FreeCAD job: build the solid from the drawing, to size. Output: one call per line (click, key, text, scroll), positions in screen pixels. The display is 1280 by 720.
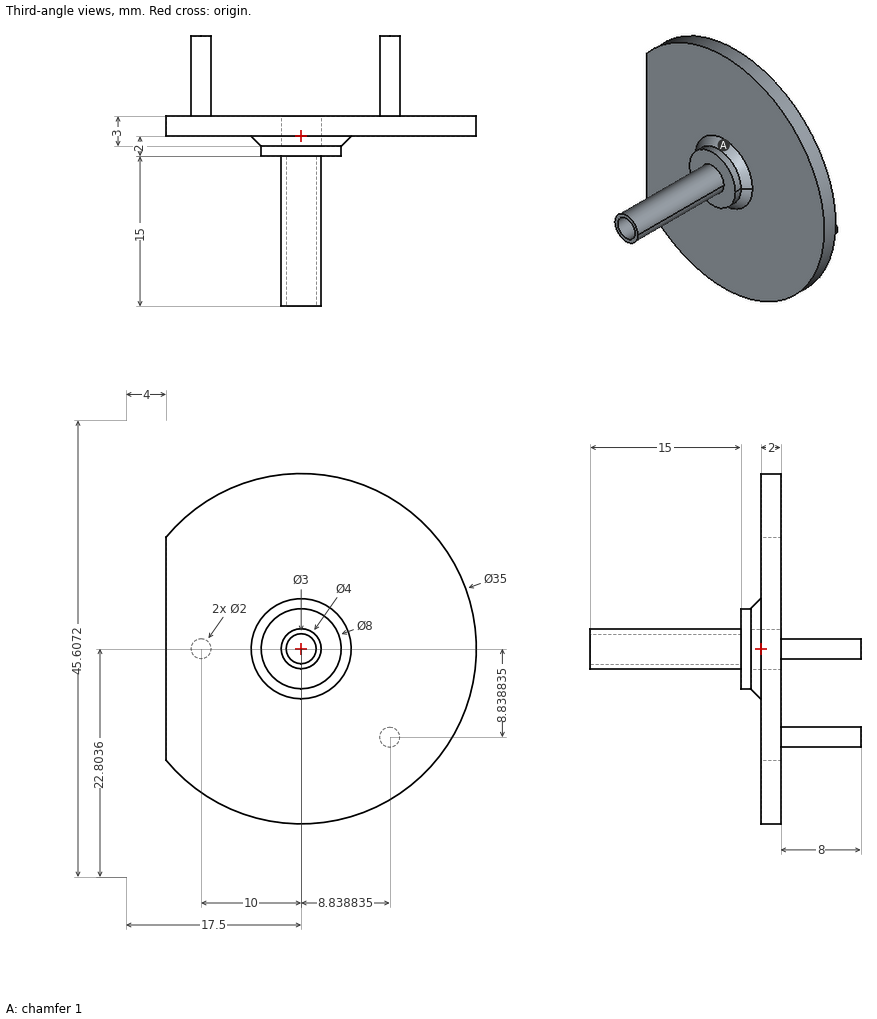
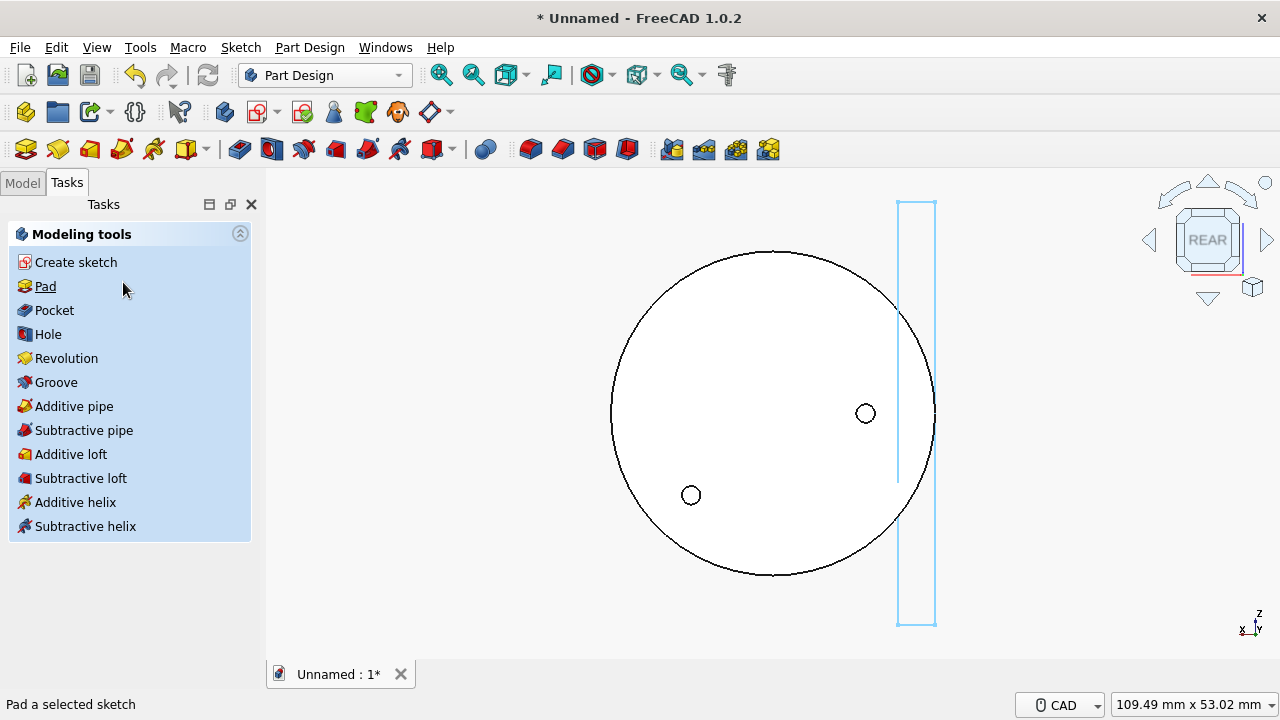
click(240, 150)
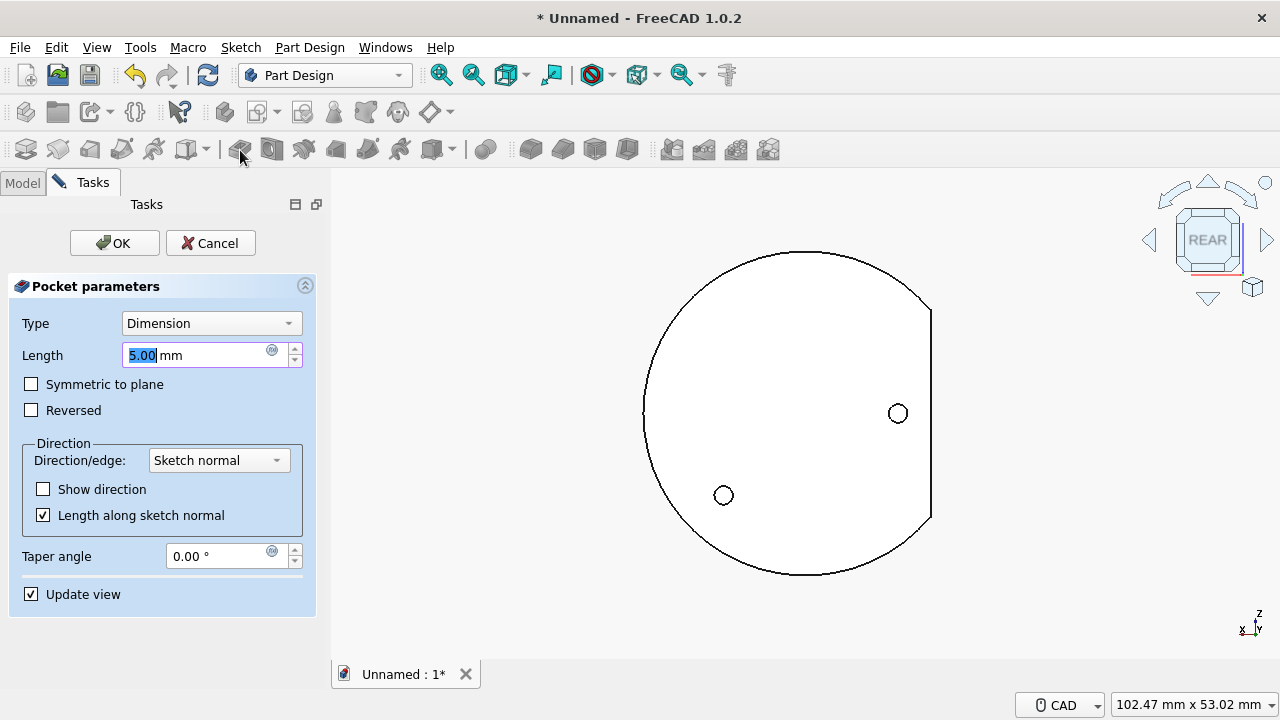
click(212, 324)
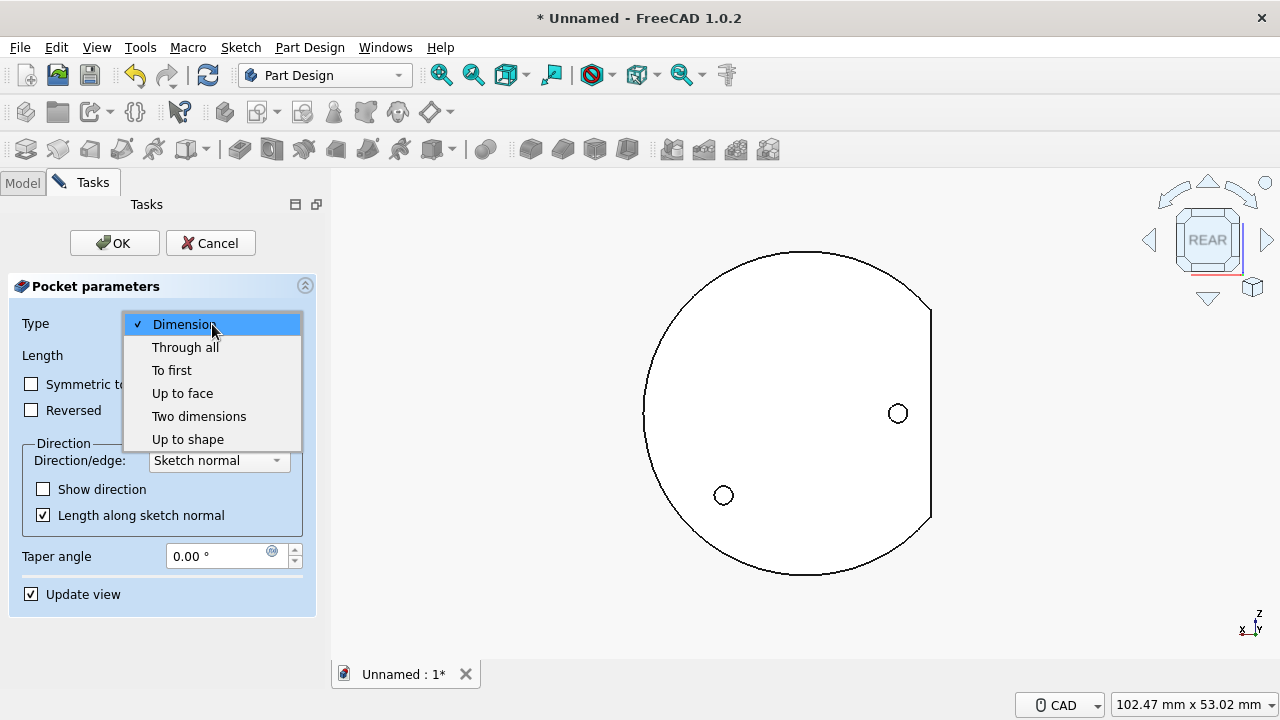
click(212, 348)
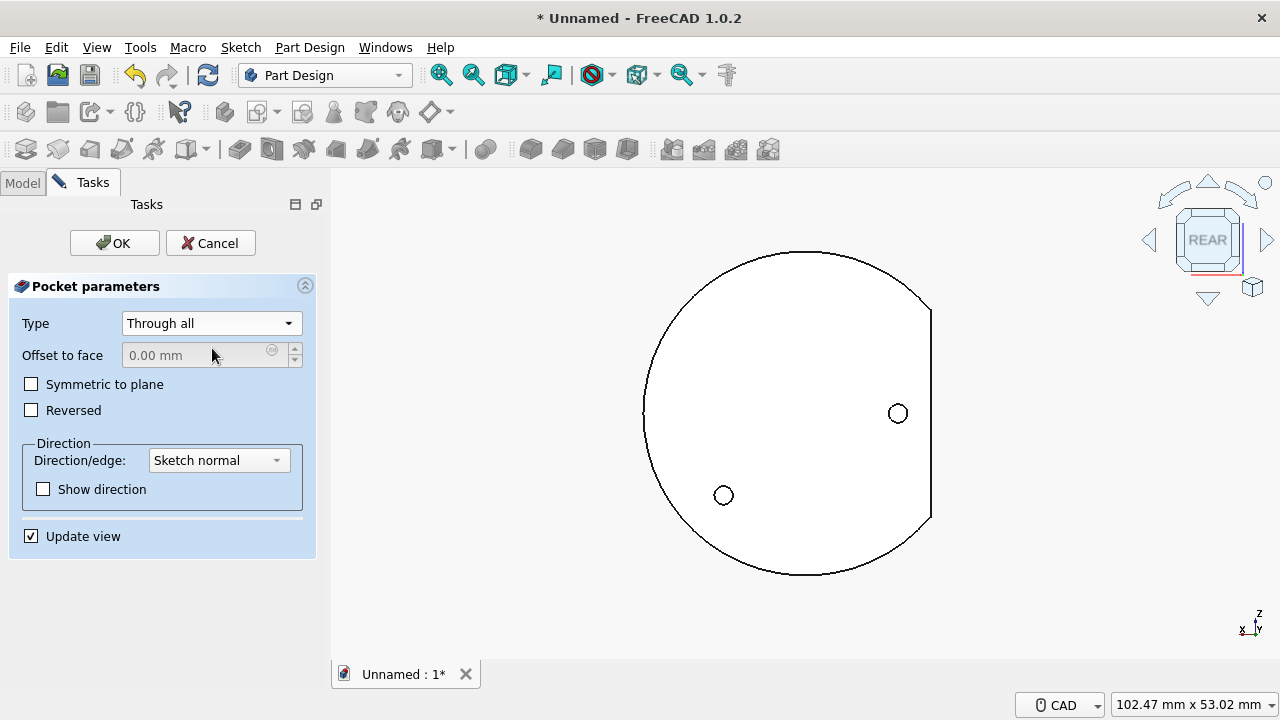
click(115, 243)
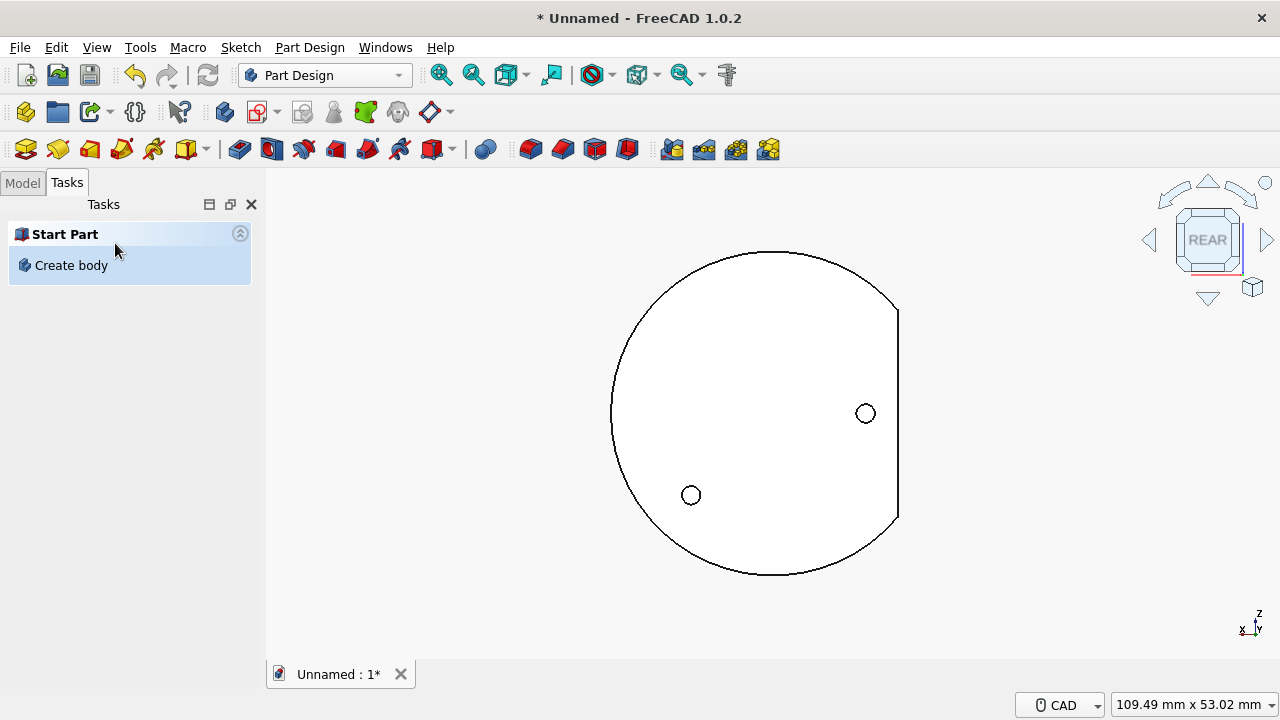
click(754, 366)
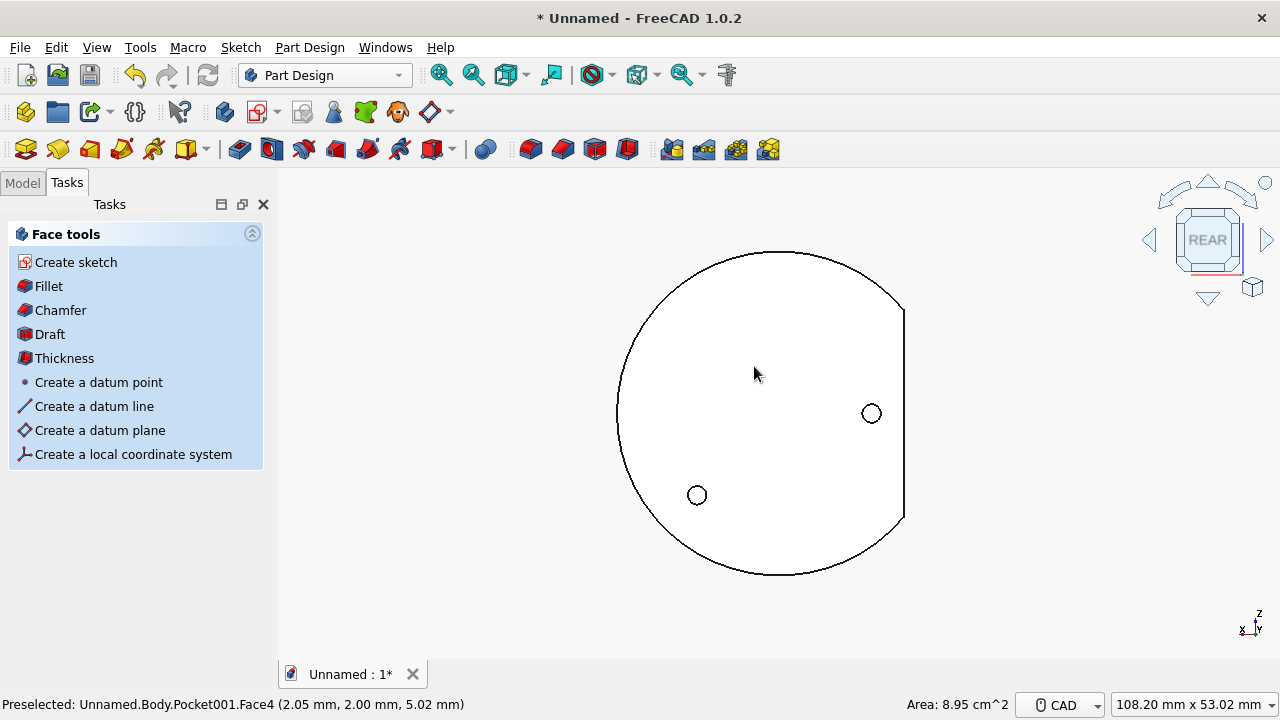
click(258, 112)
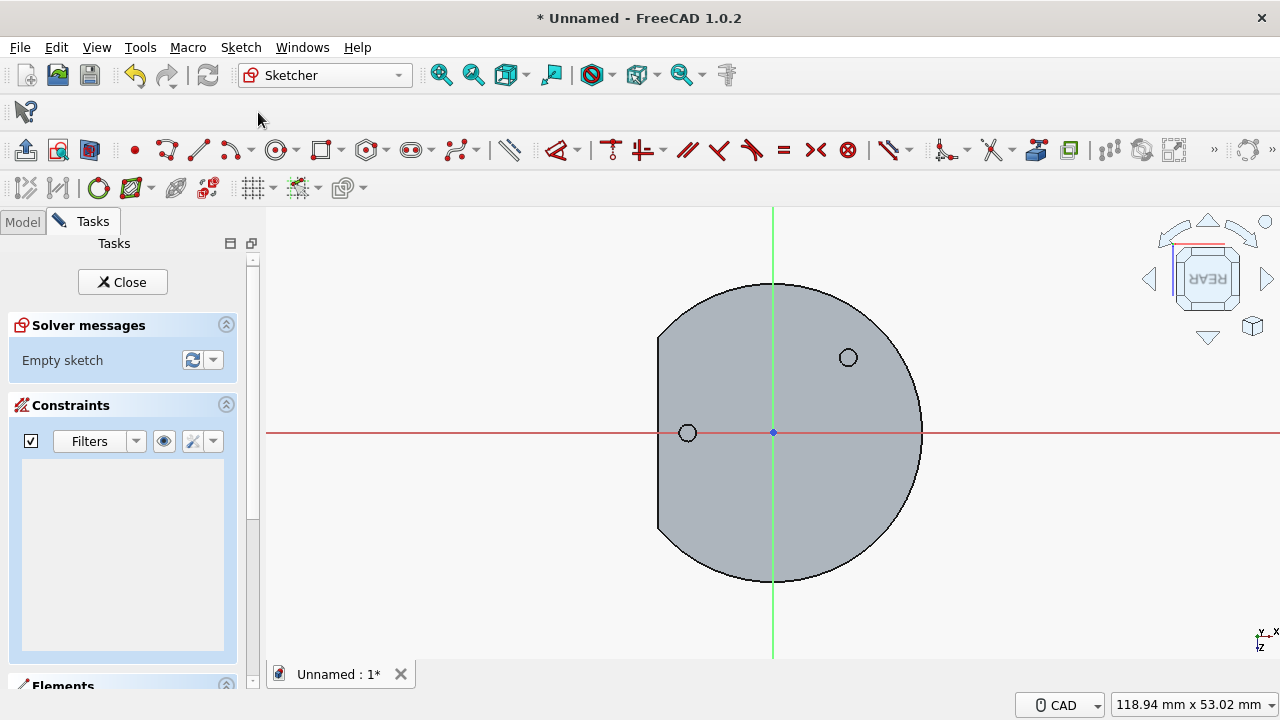
click(90, 150)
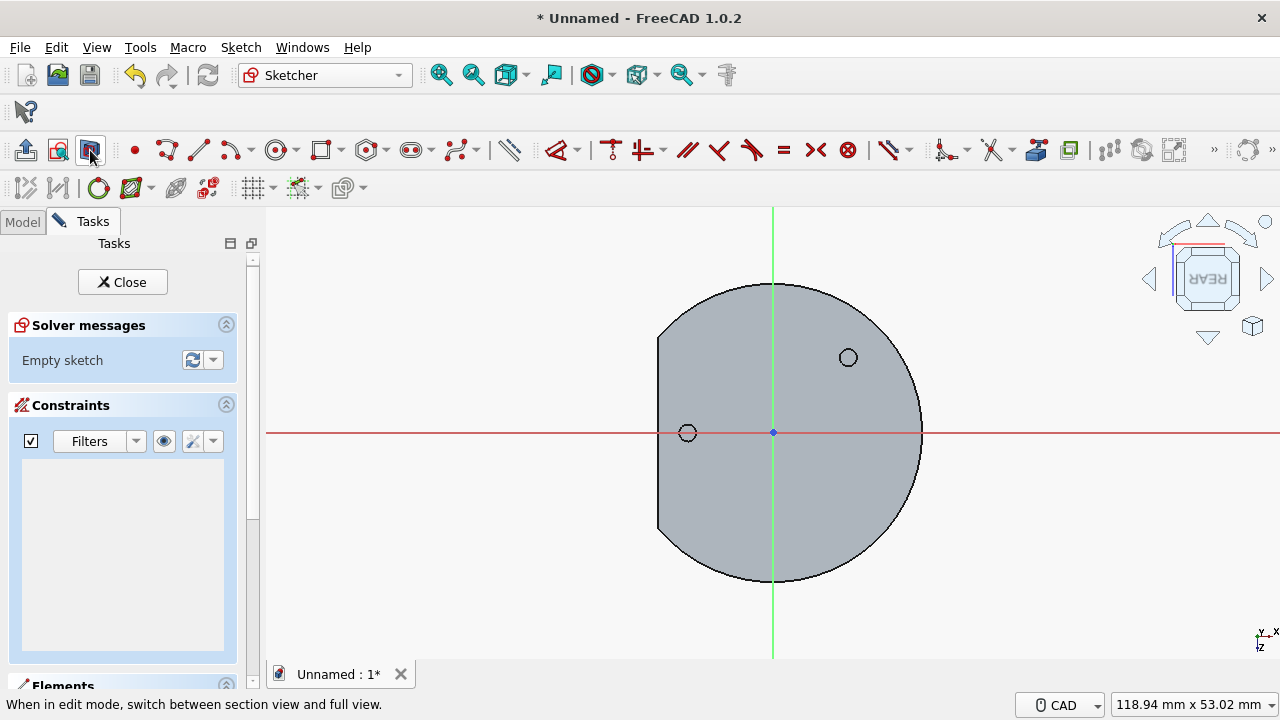
scroll(782, 433, up, 11)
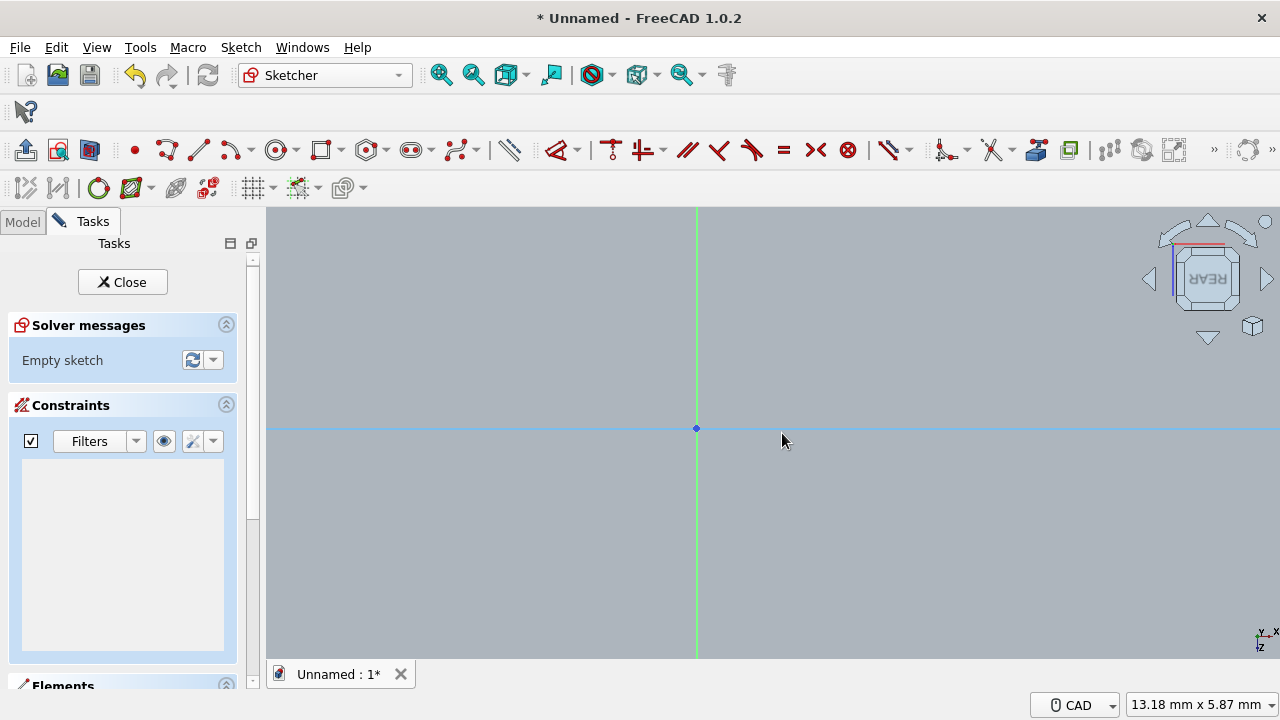
click(276, 150)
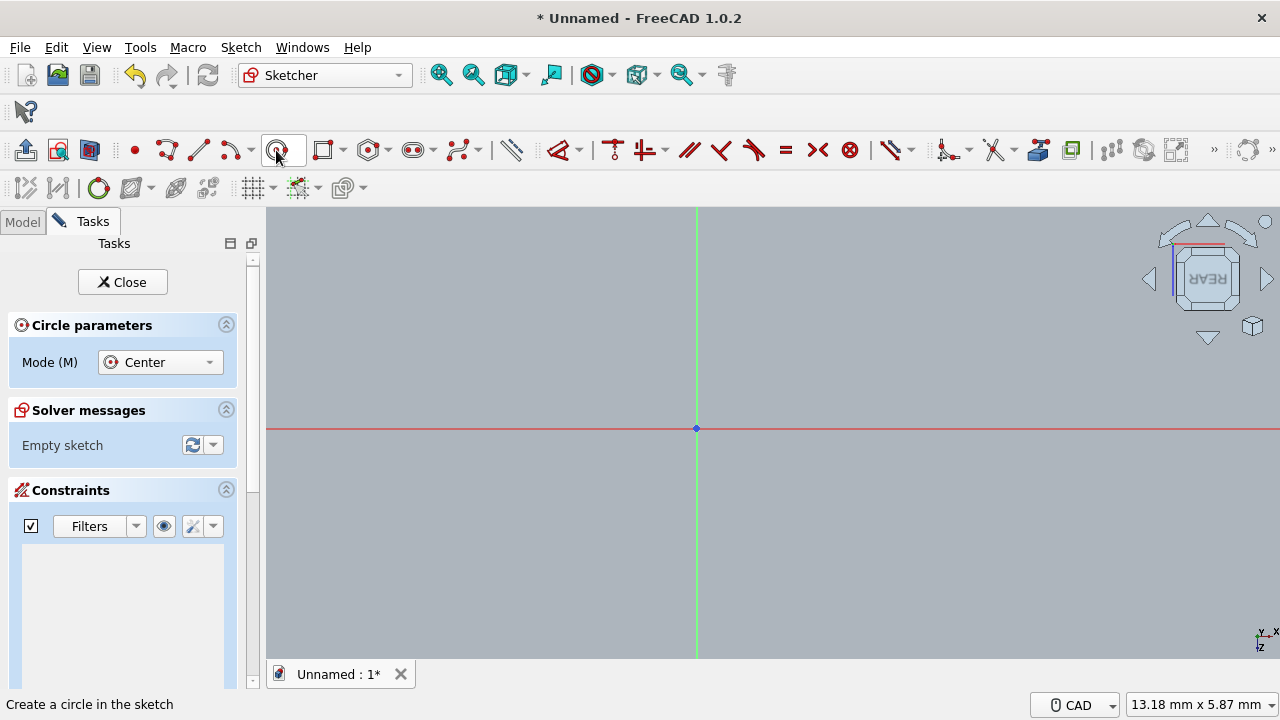
click(697, 429)
click(805, 320)
key(Escape)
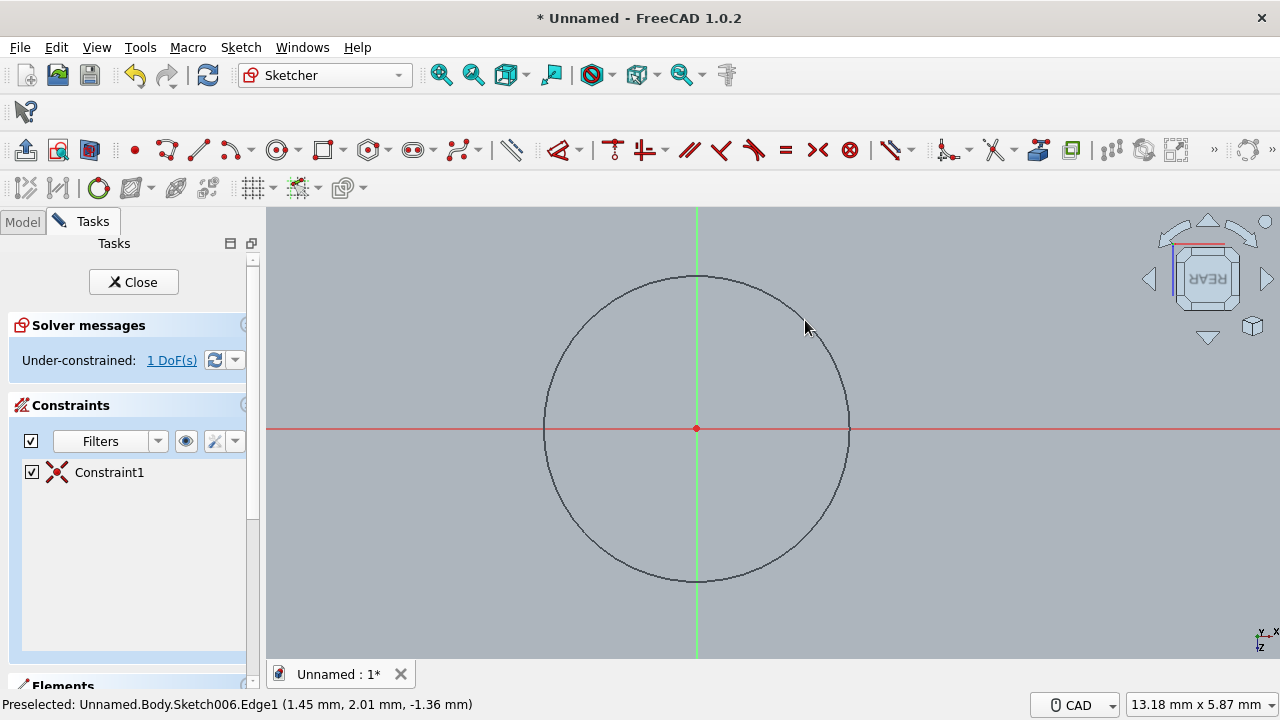
click(558, 150)